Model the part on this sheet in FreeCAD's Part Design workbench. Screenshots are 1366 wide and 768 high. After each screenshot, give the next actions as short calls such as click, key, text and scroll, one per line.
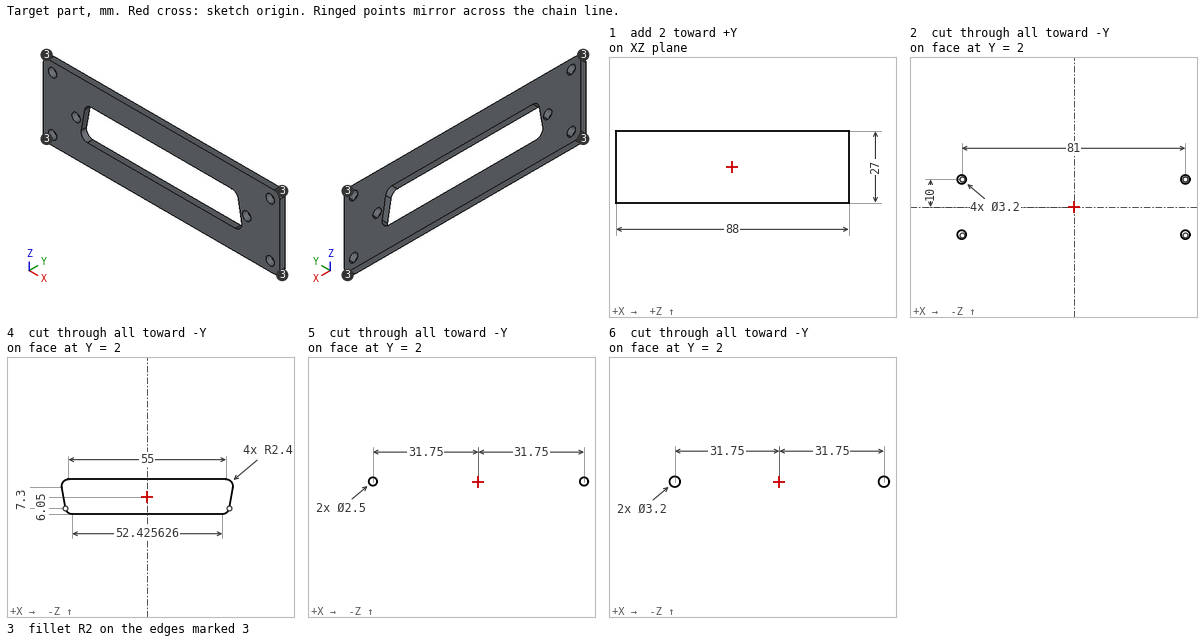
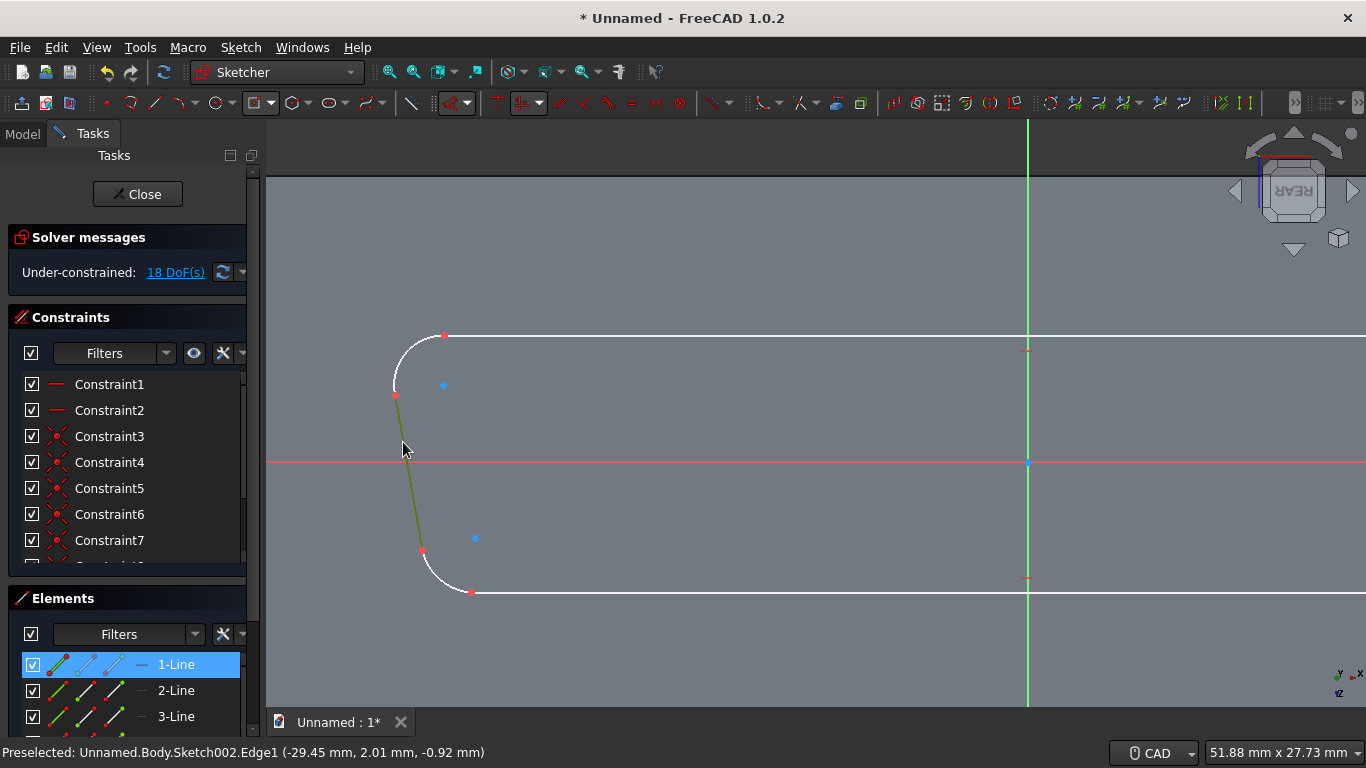
click(431, 569)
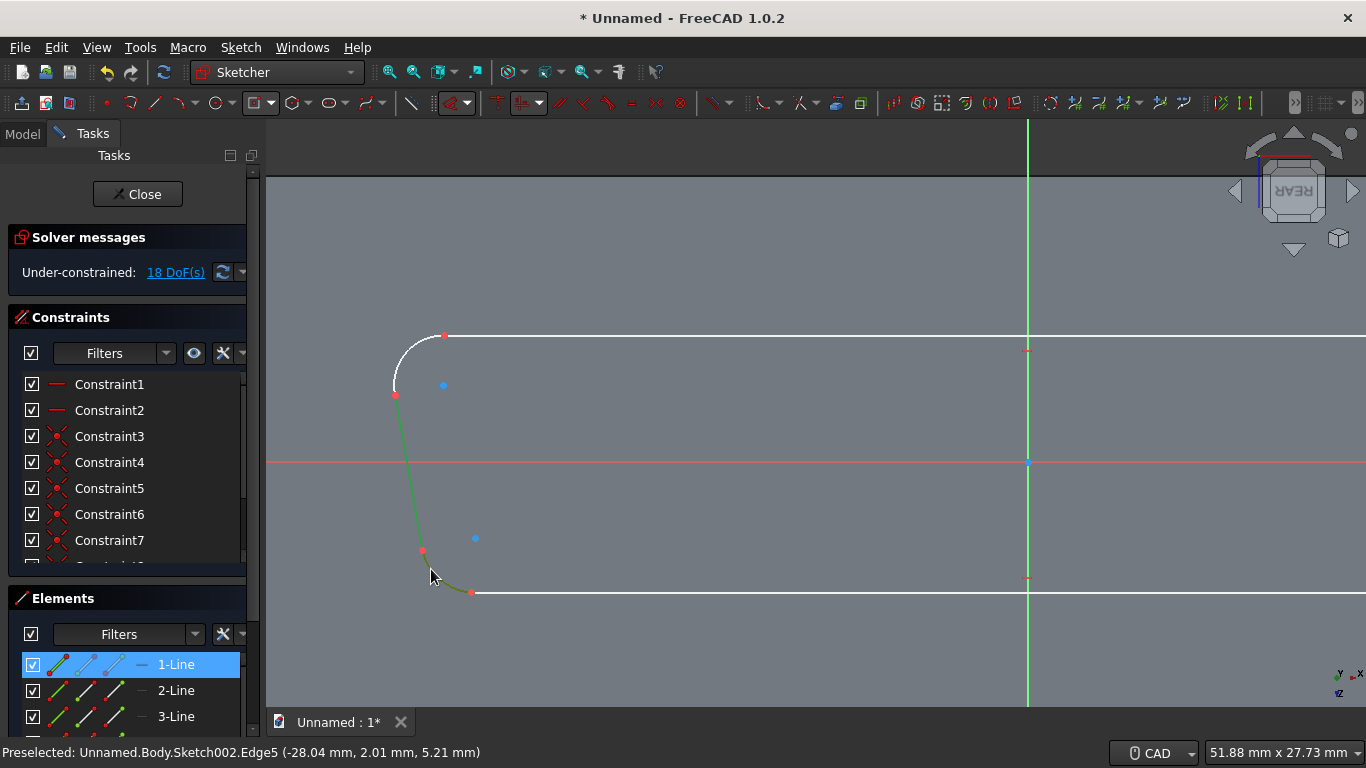
click(608, 104)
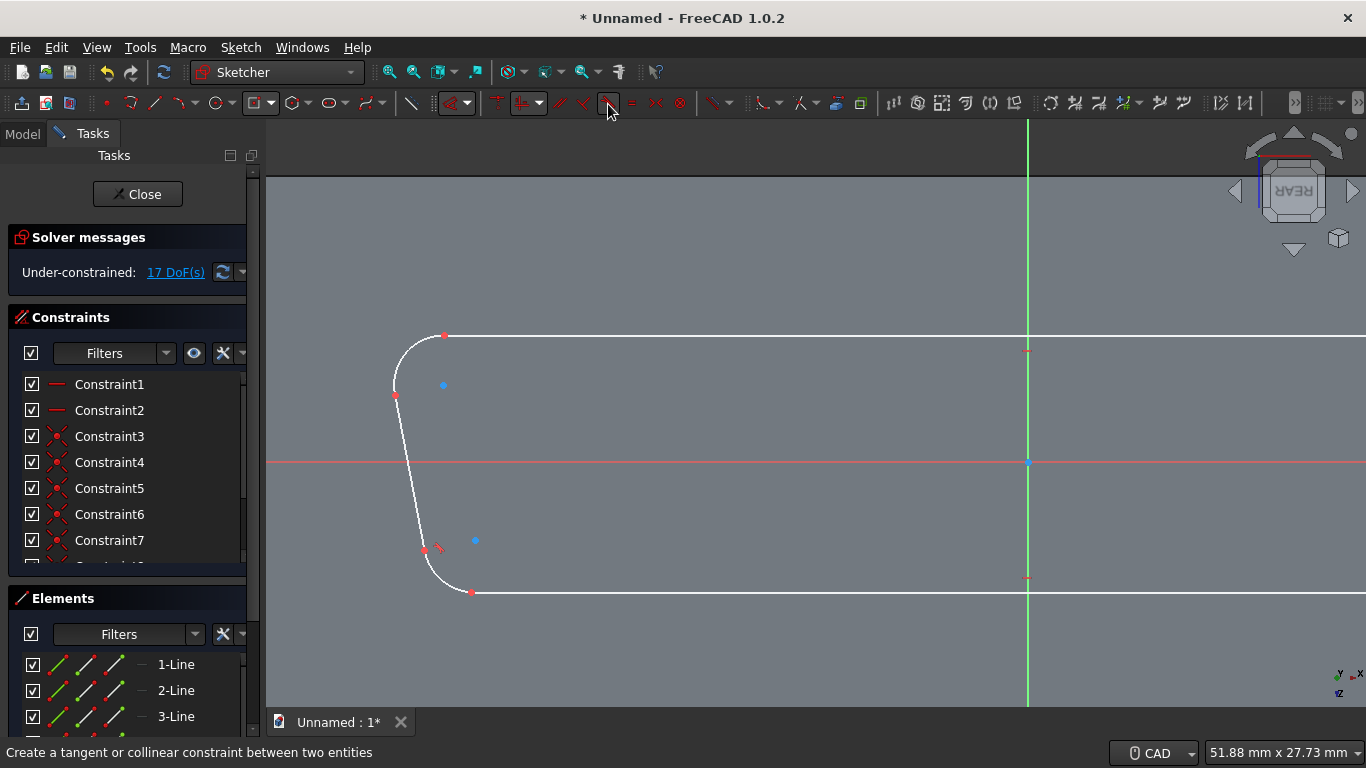
click(404, 442)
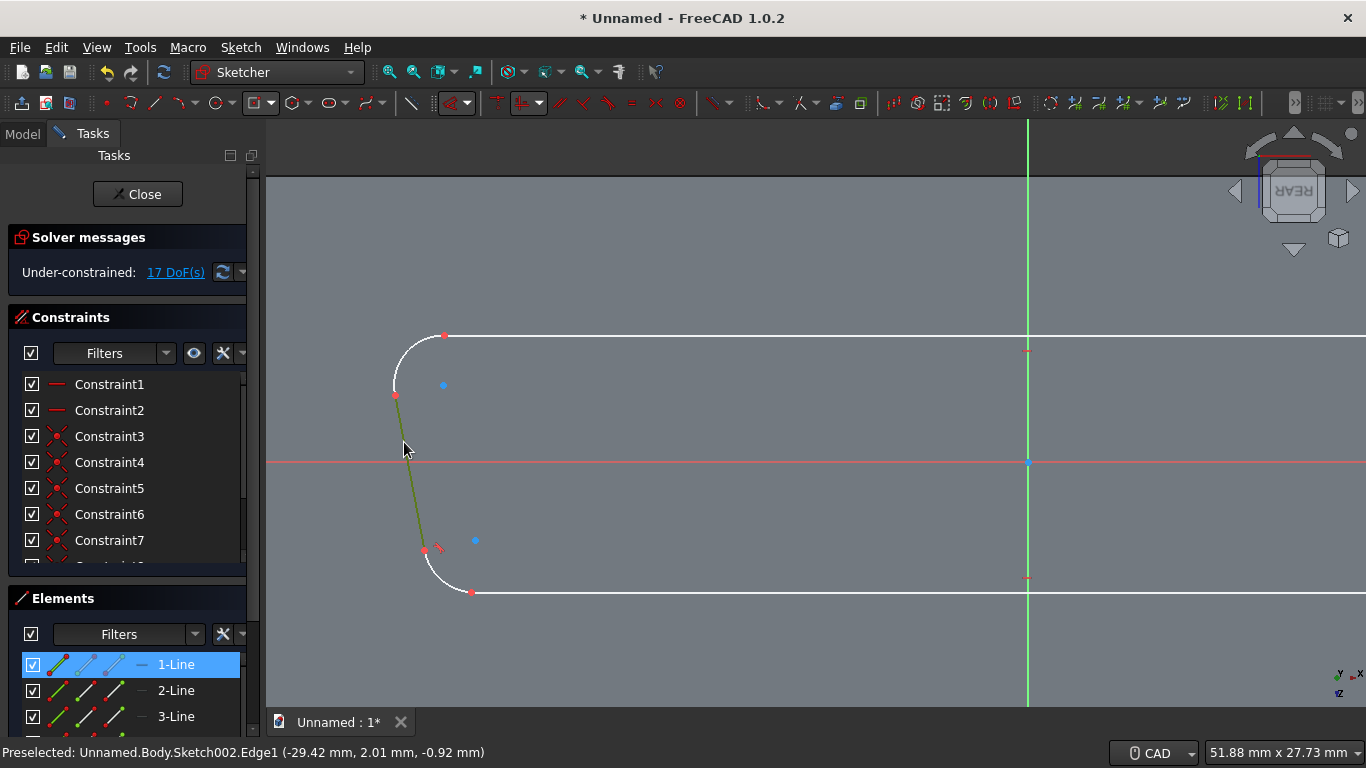
click(419, 342)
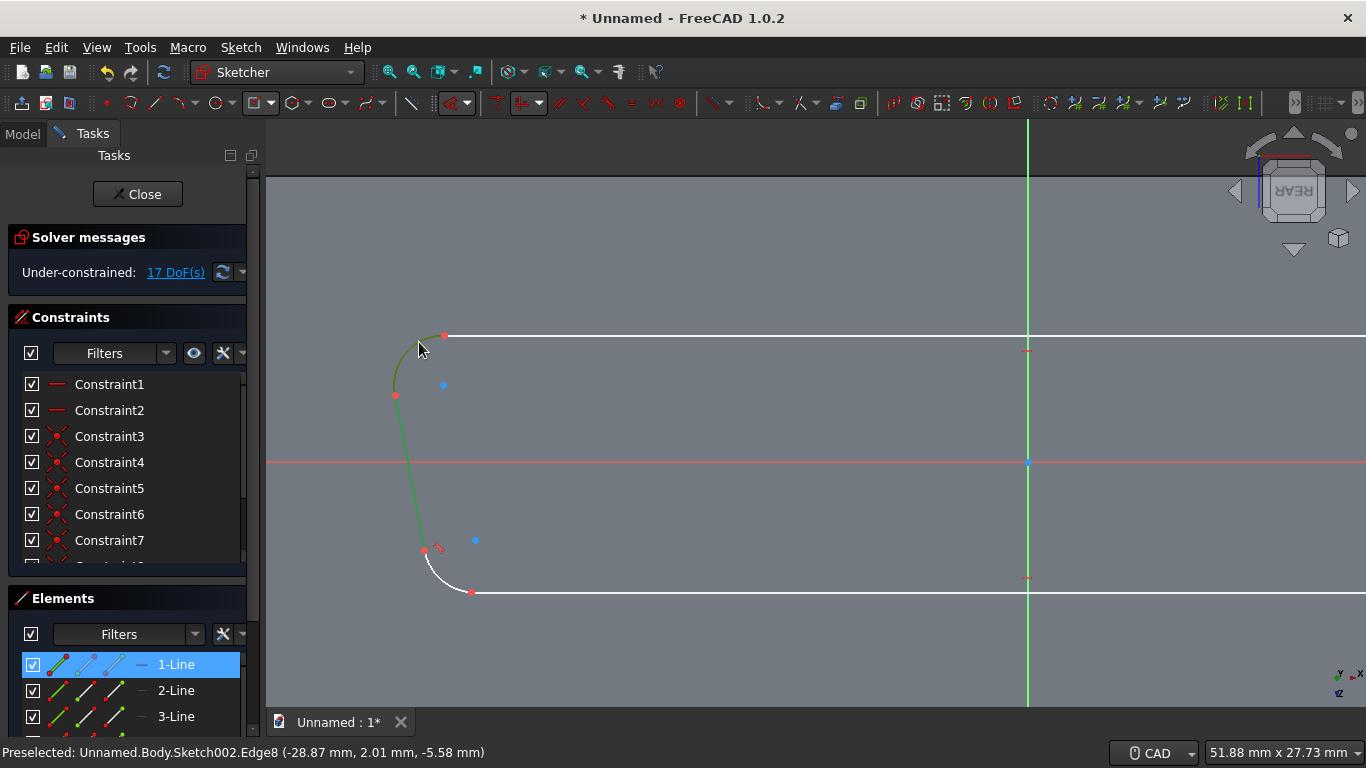
click(608, 104)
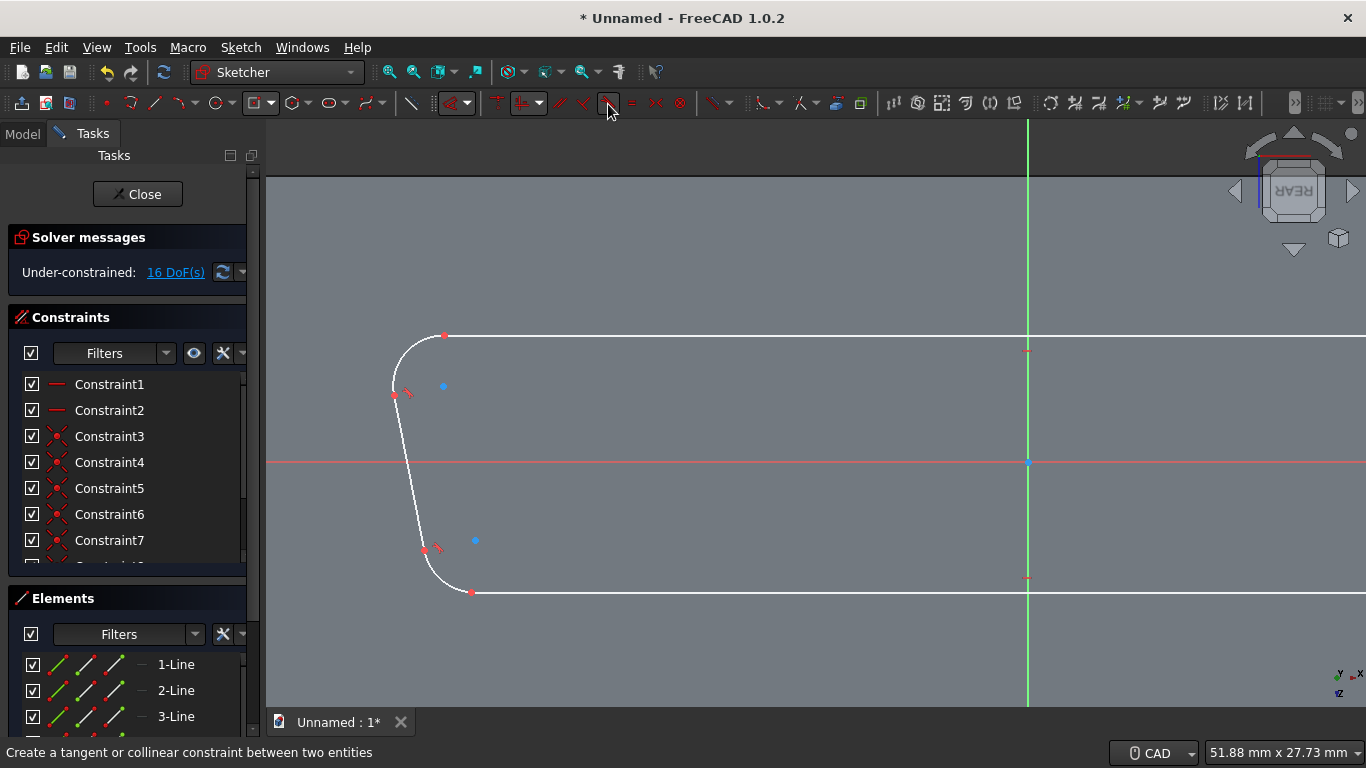
click(805, 593)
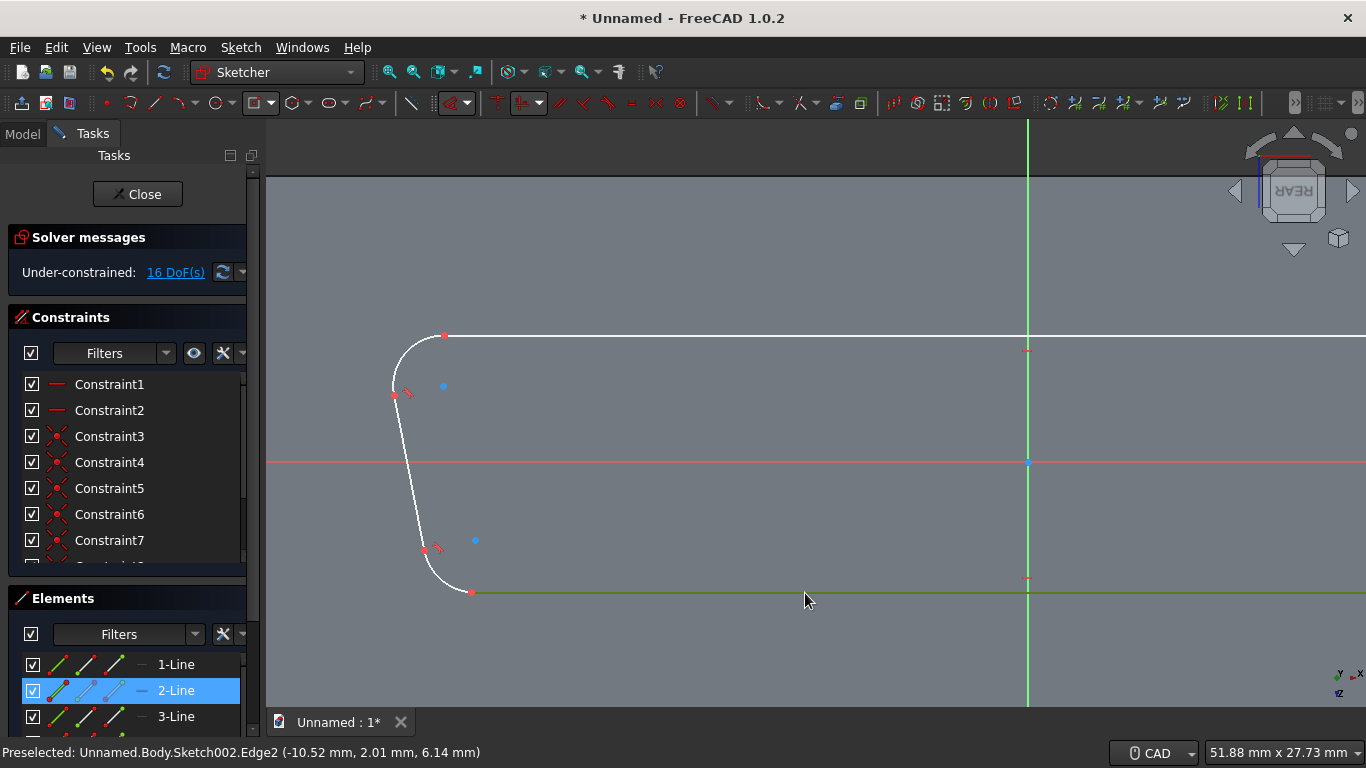
click(432, 569)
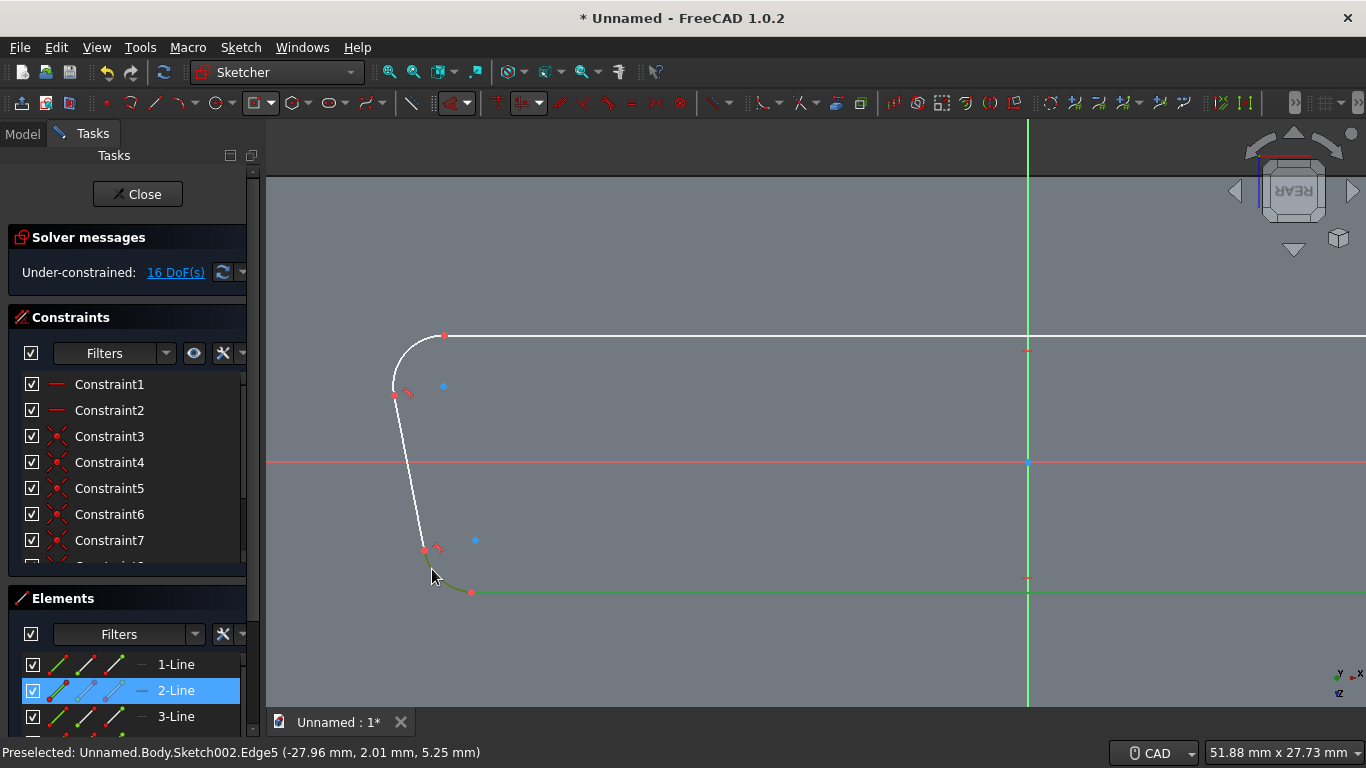
click(608, 104)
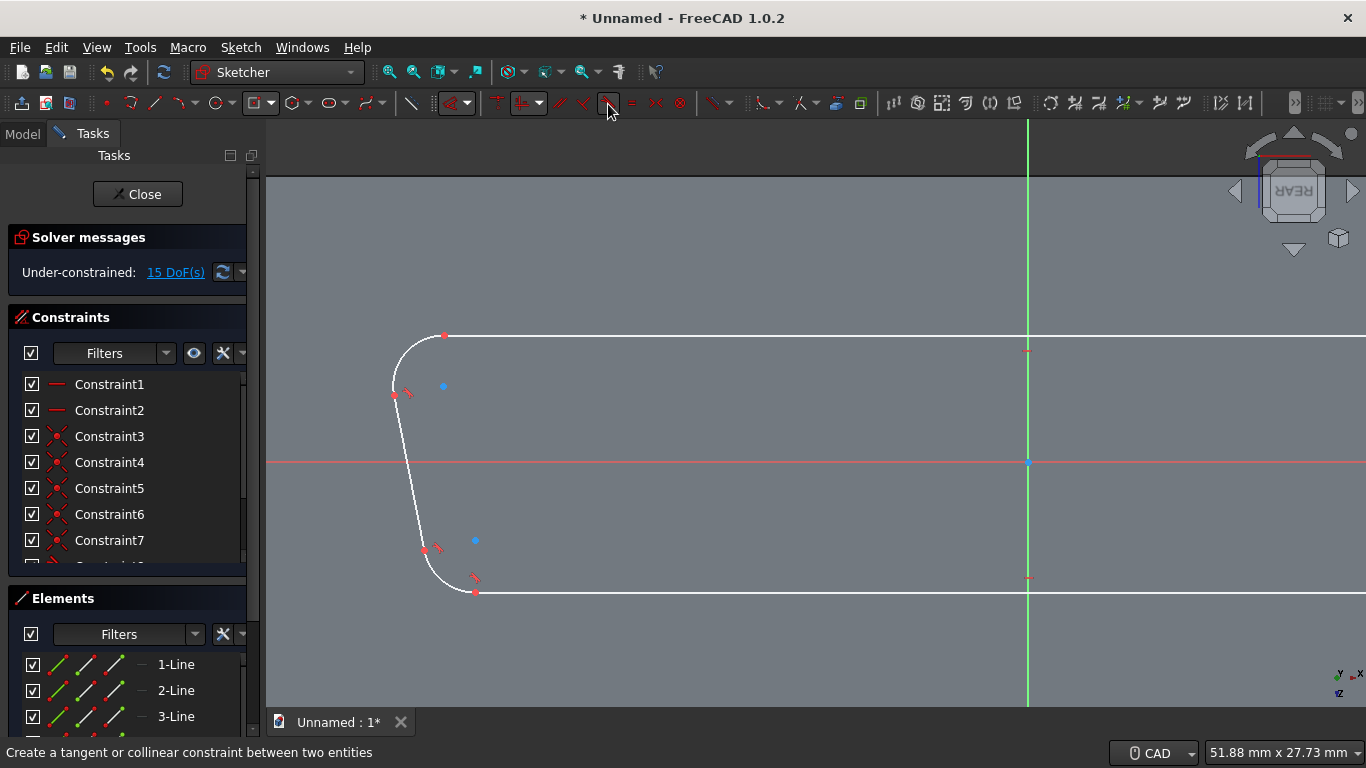
click(808, 593)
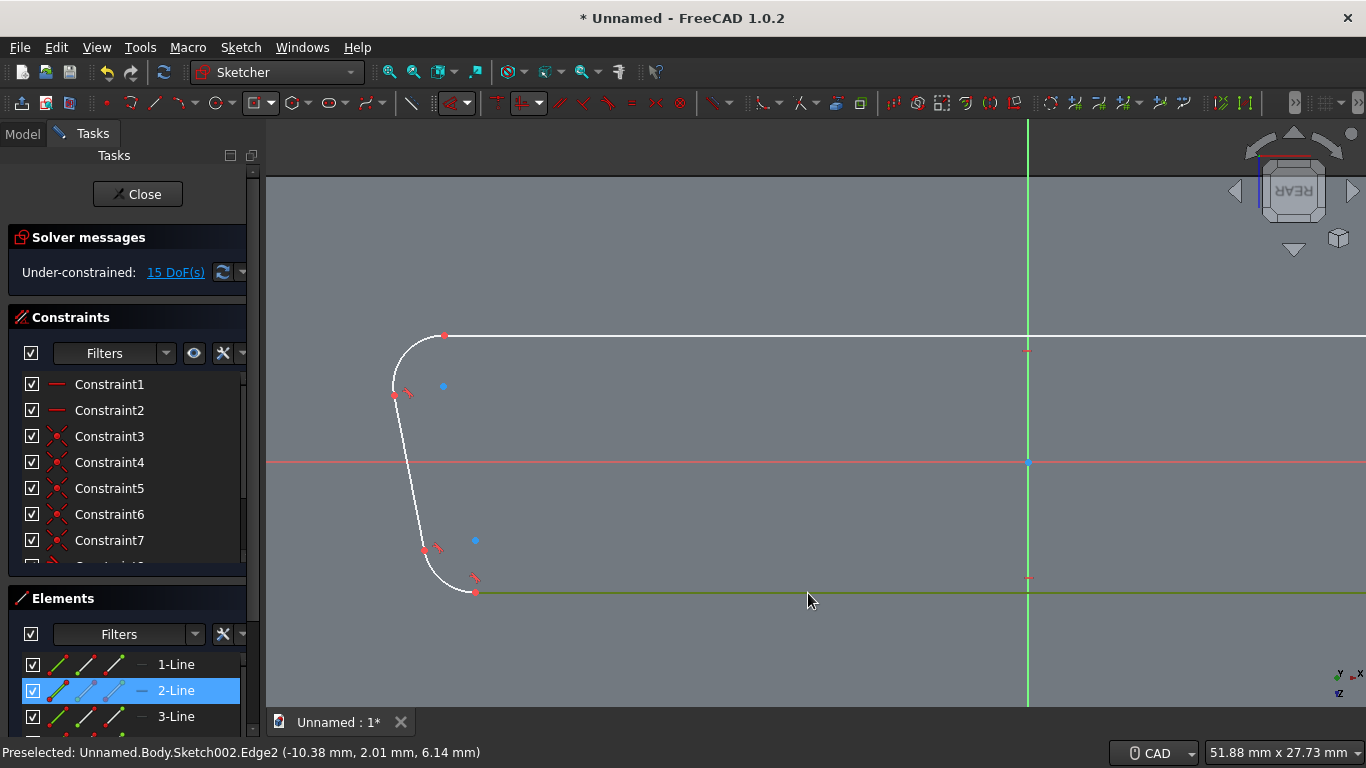
scroll(406, 353, down, 3)